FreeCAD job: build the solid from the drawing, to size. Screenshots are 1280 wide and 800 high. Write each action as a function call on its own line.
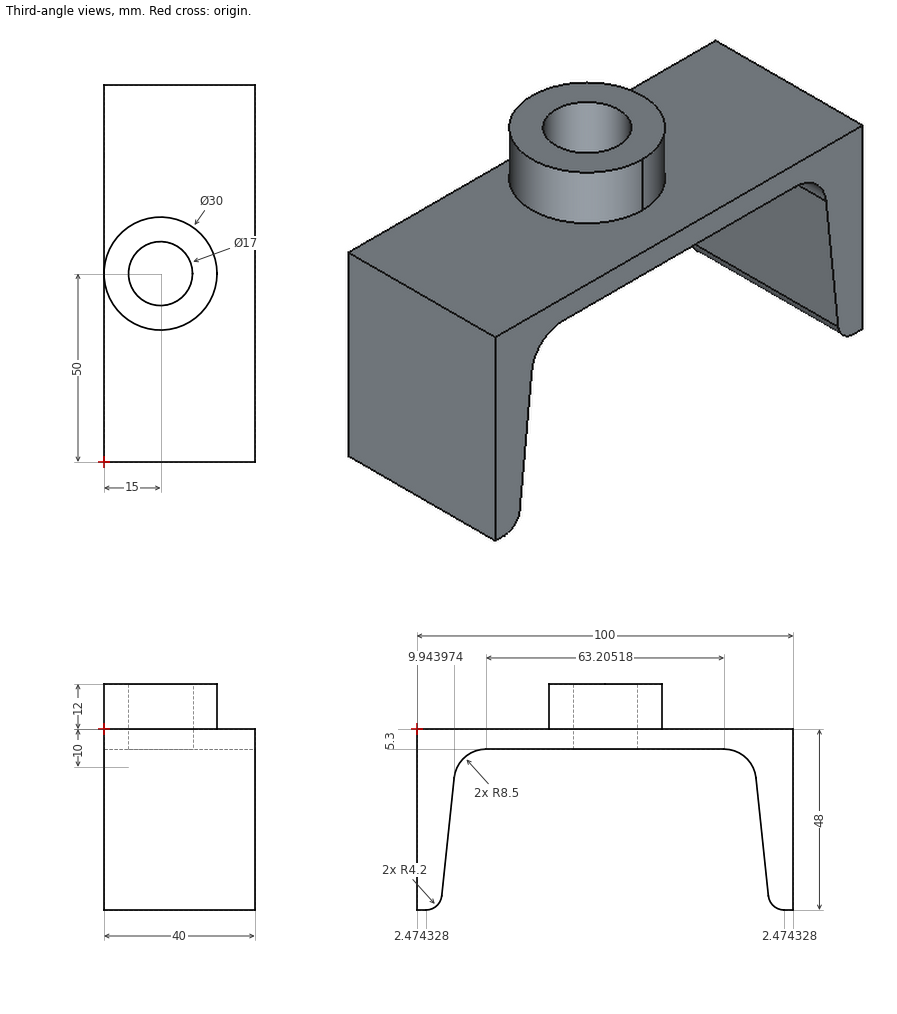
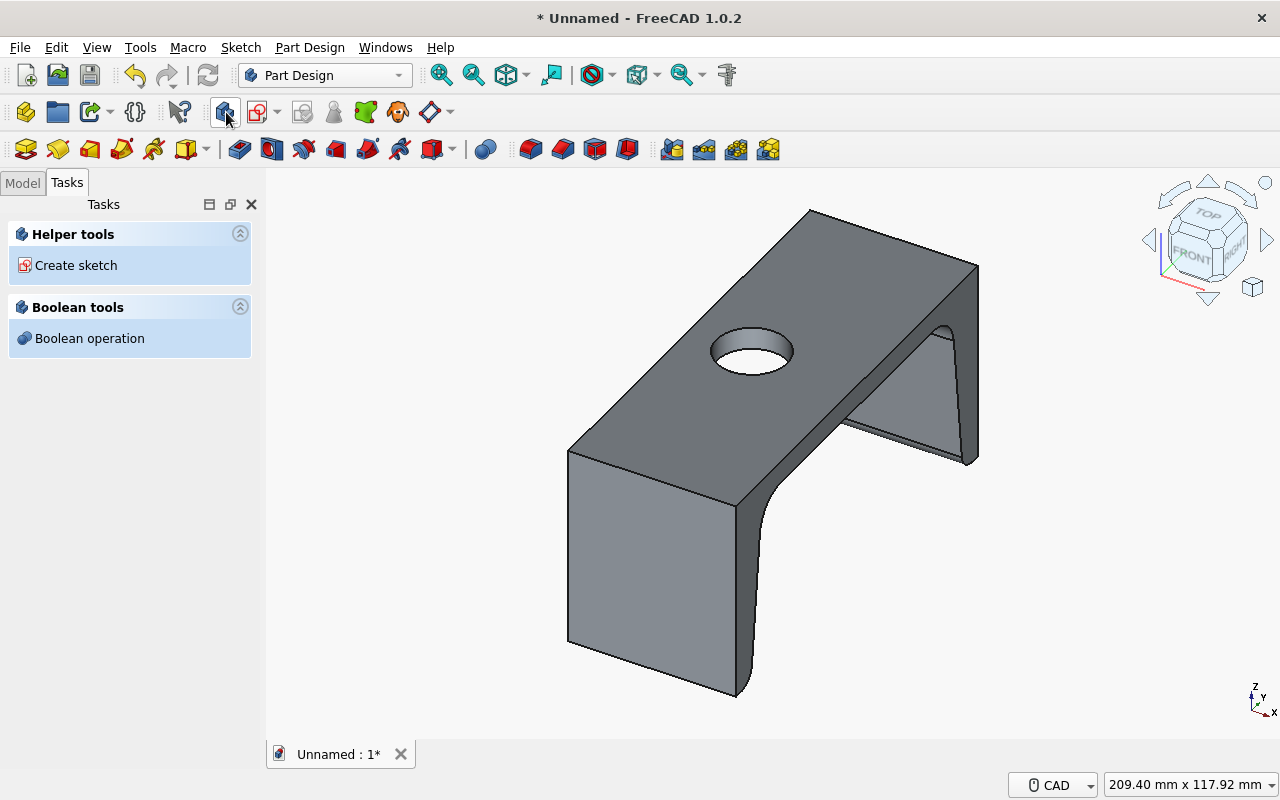
click(306, 699)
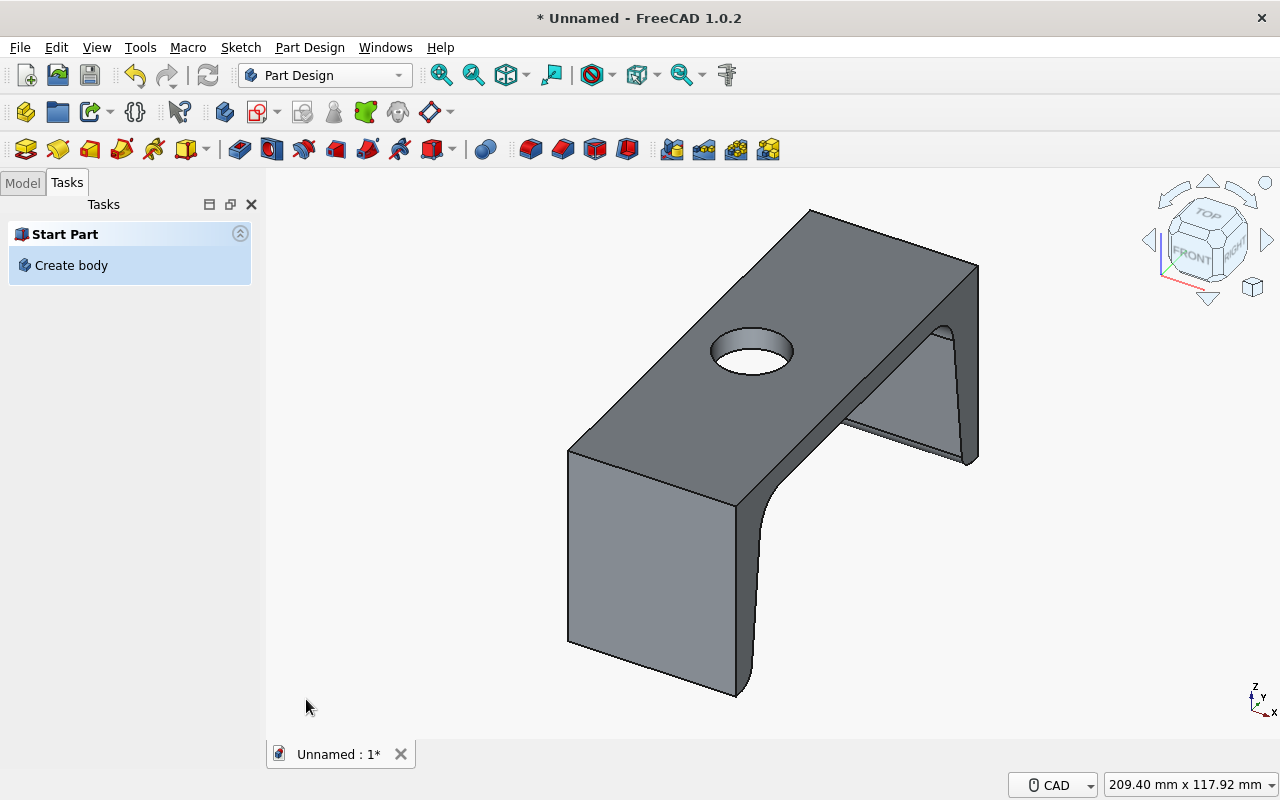
click(258, 112)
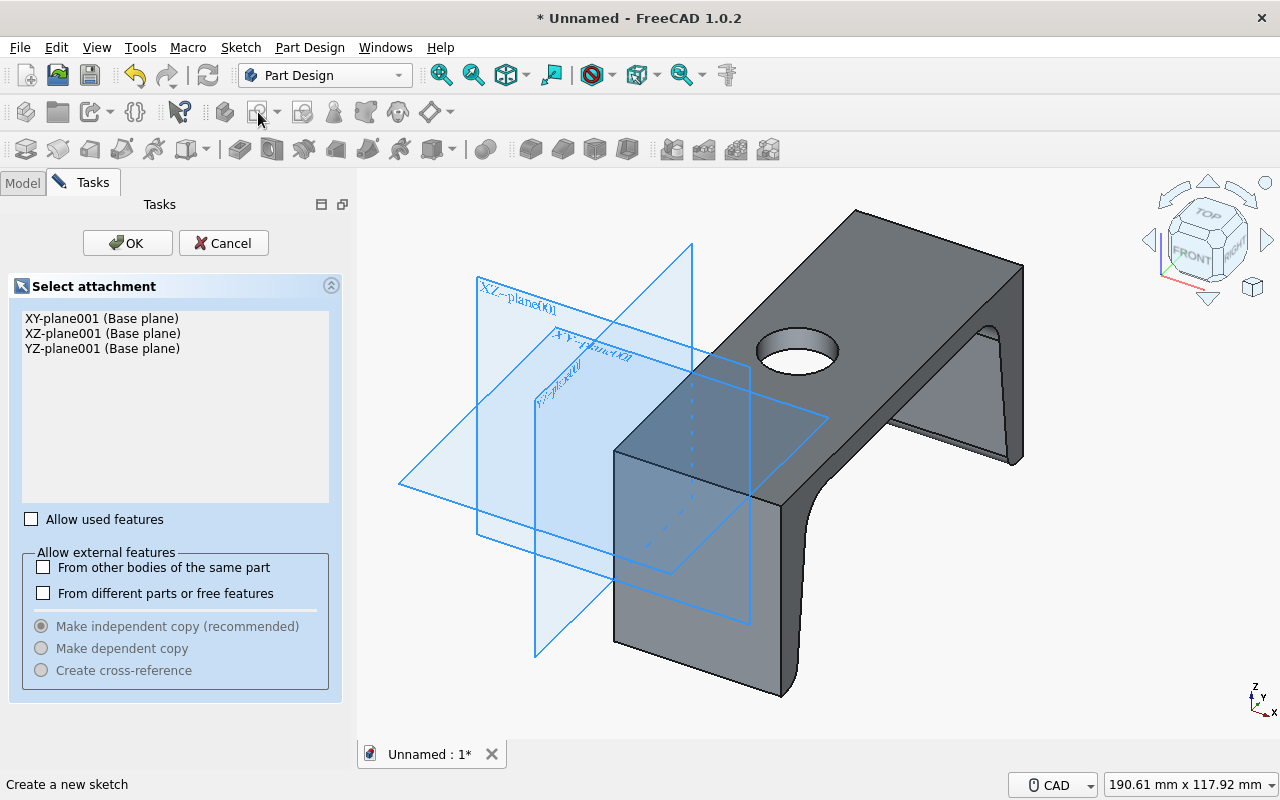
click(82, 318)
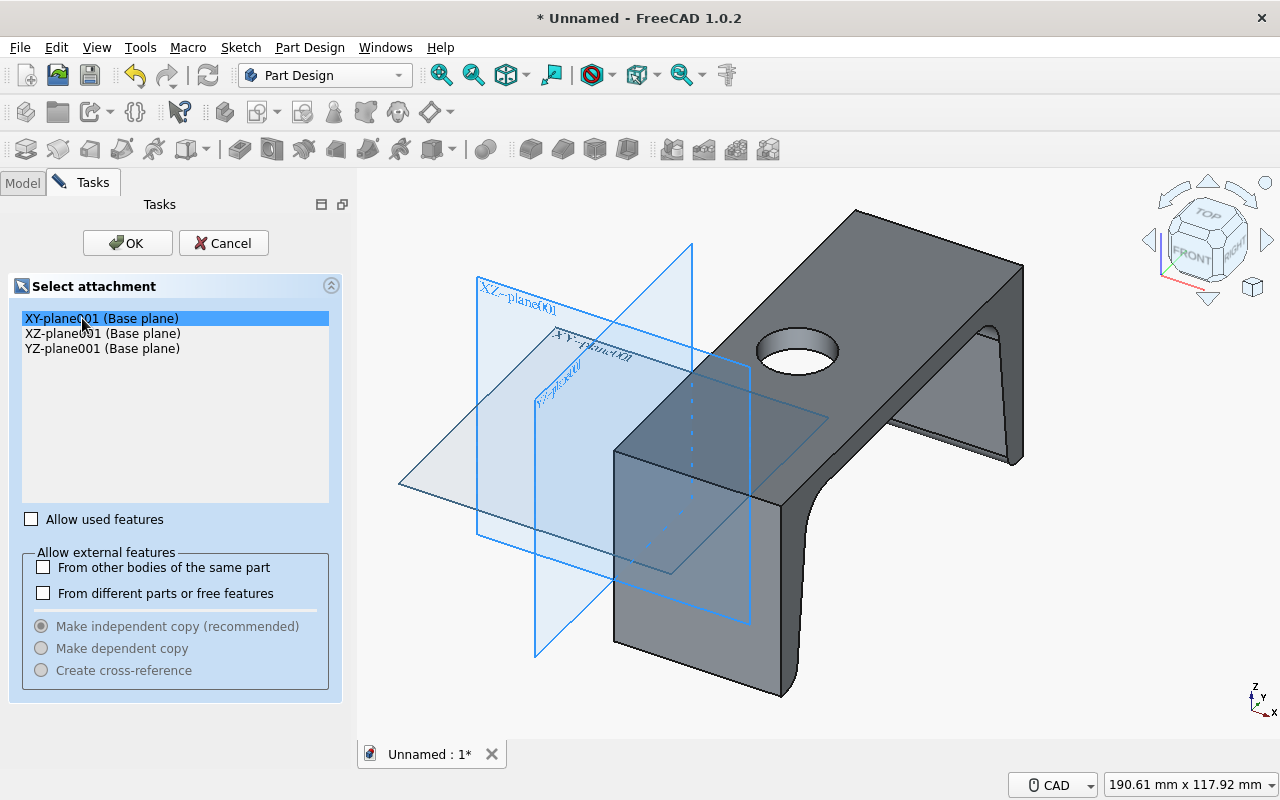
click(128, 243)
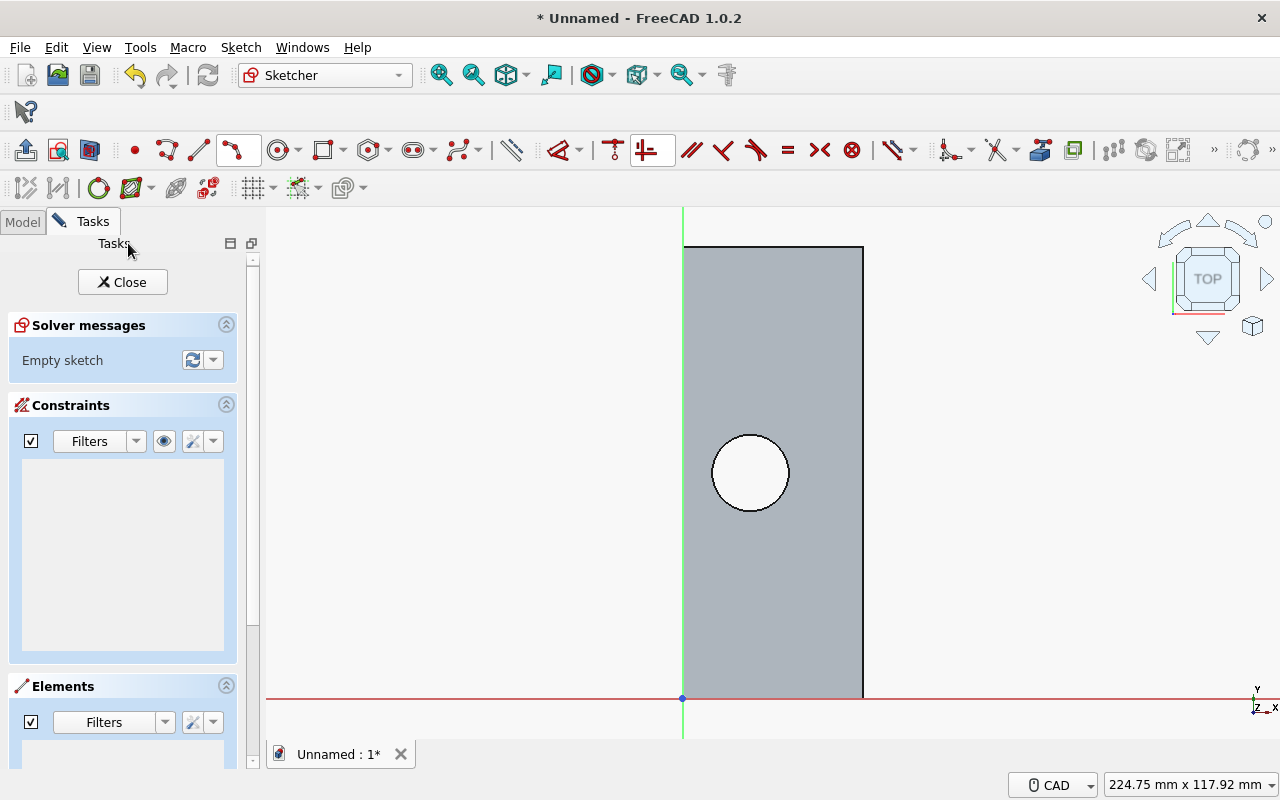
scroll(497, 235, down, 1)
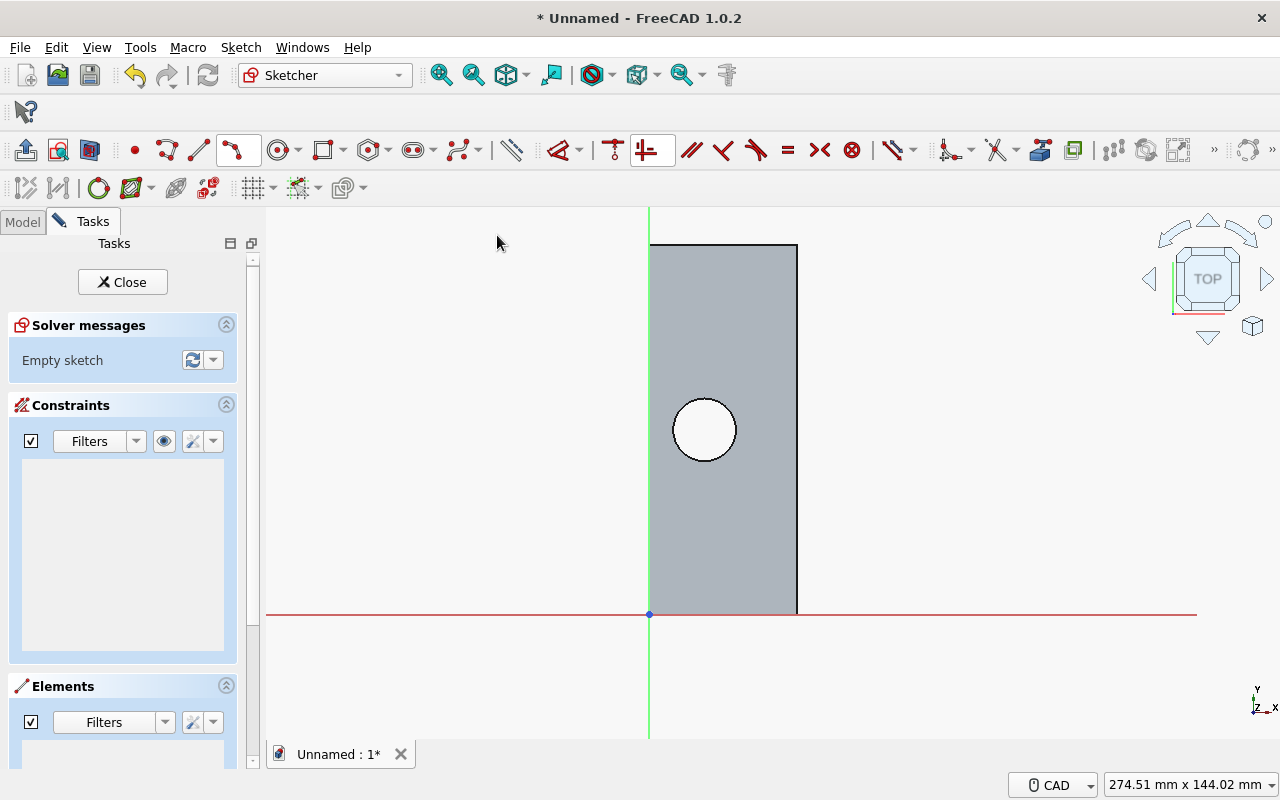
scroll(705, 538, up, 2)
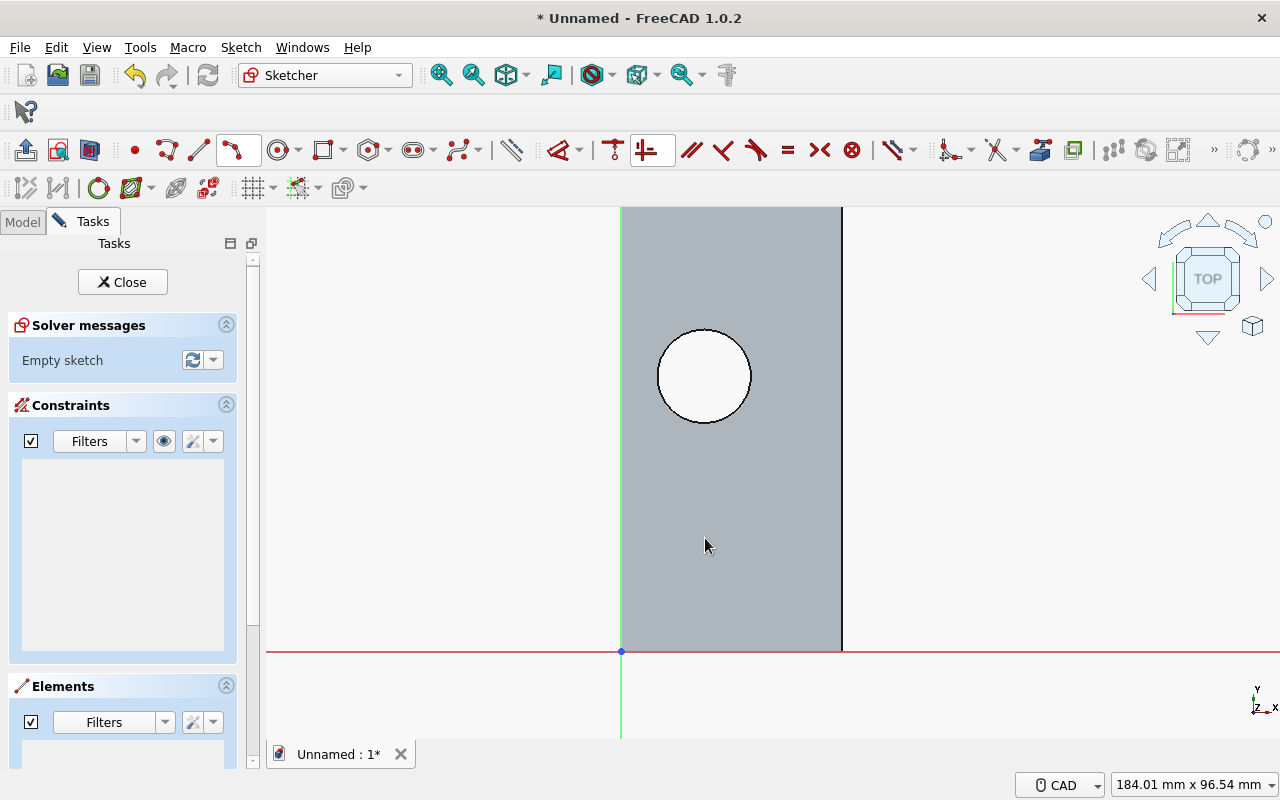
click(278, 150)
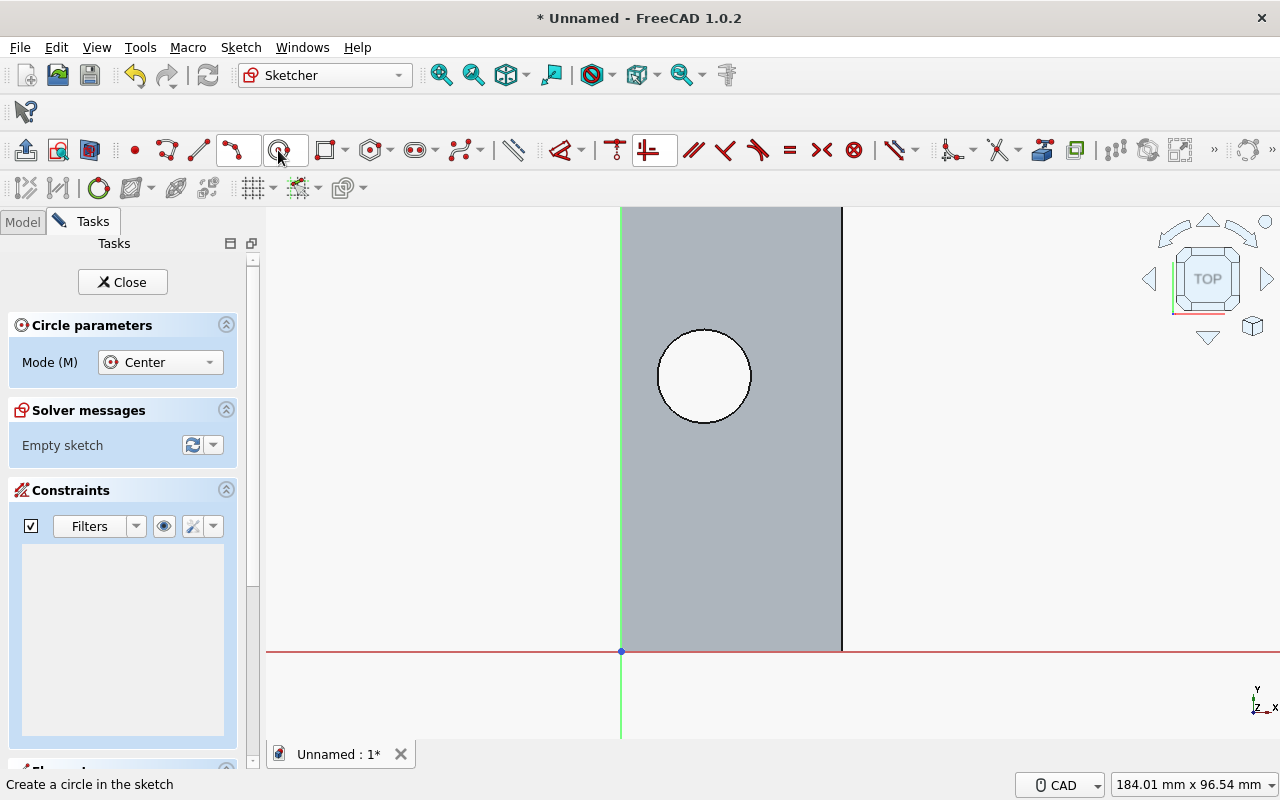
click(704, 376)
move(763, 318)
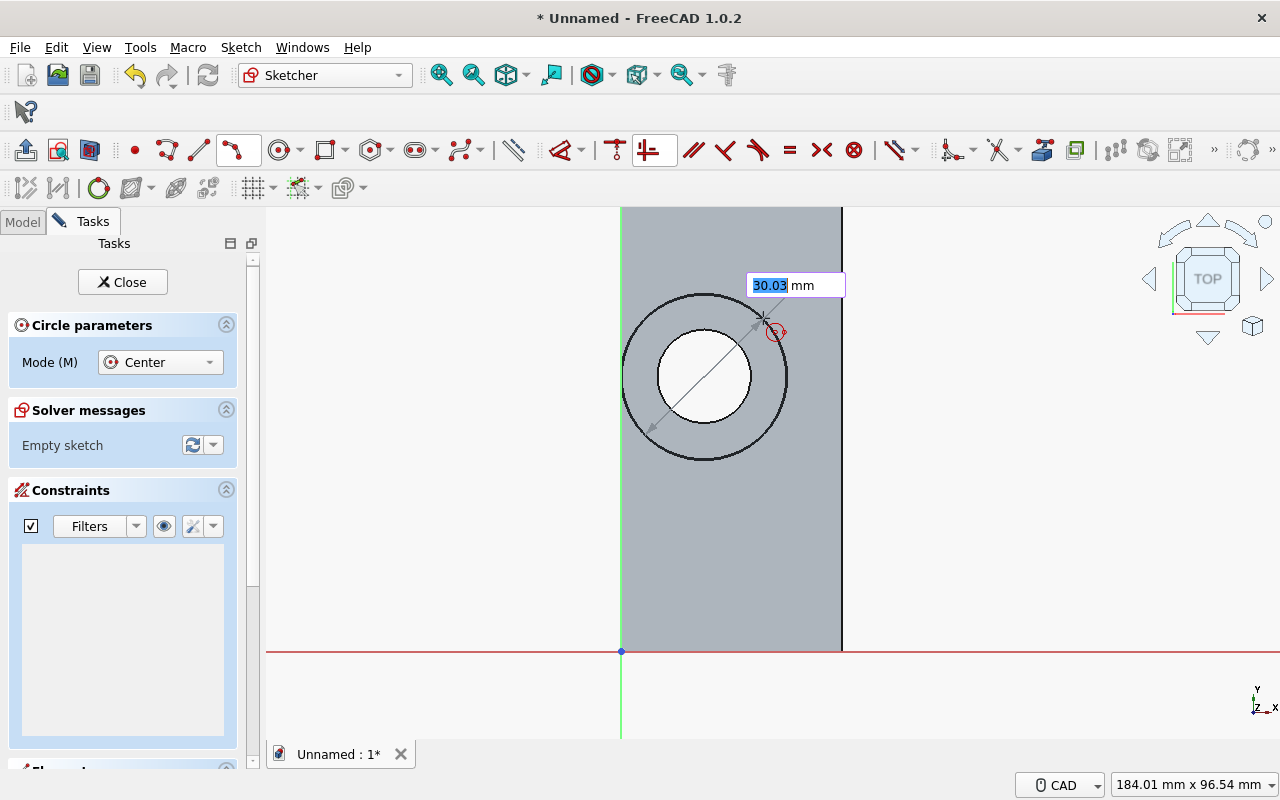
text(30)
key(Return)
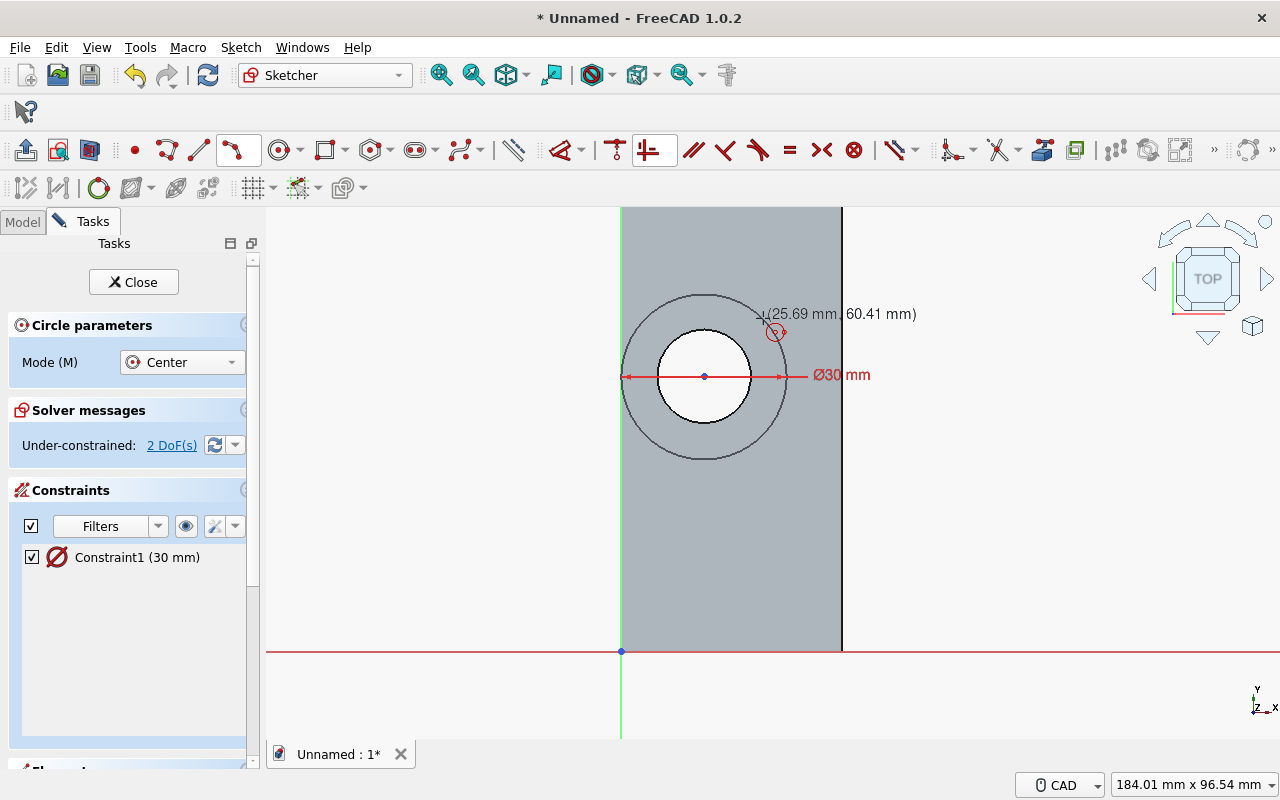
click(704, 377)
move(737, 343)